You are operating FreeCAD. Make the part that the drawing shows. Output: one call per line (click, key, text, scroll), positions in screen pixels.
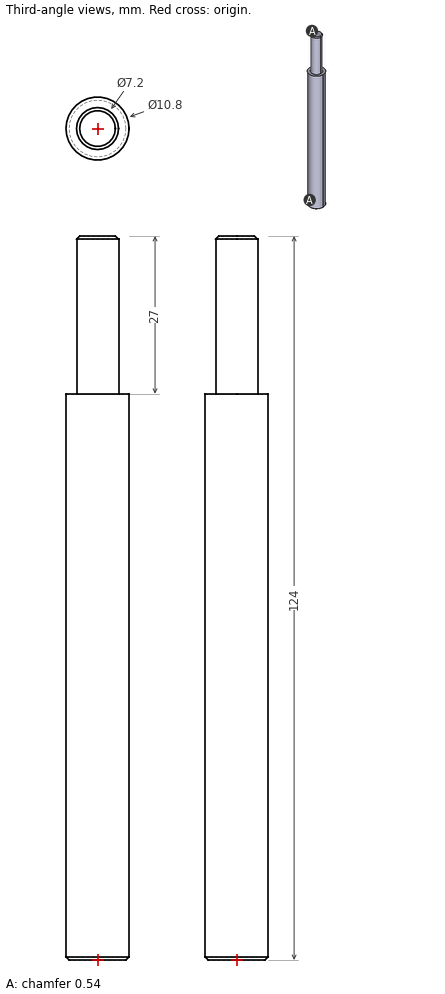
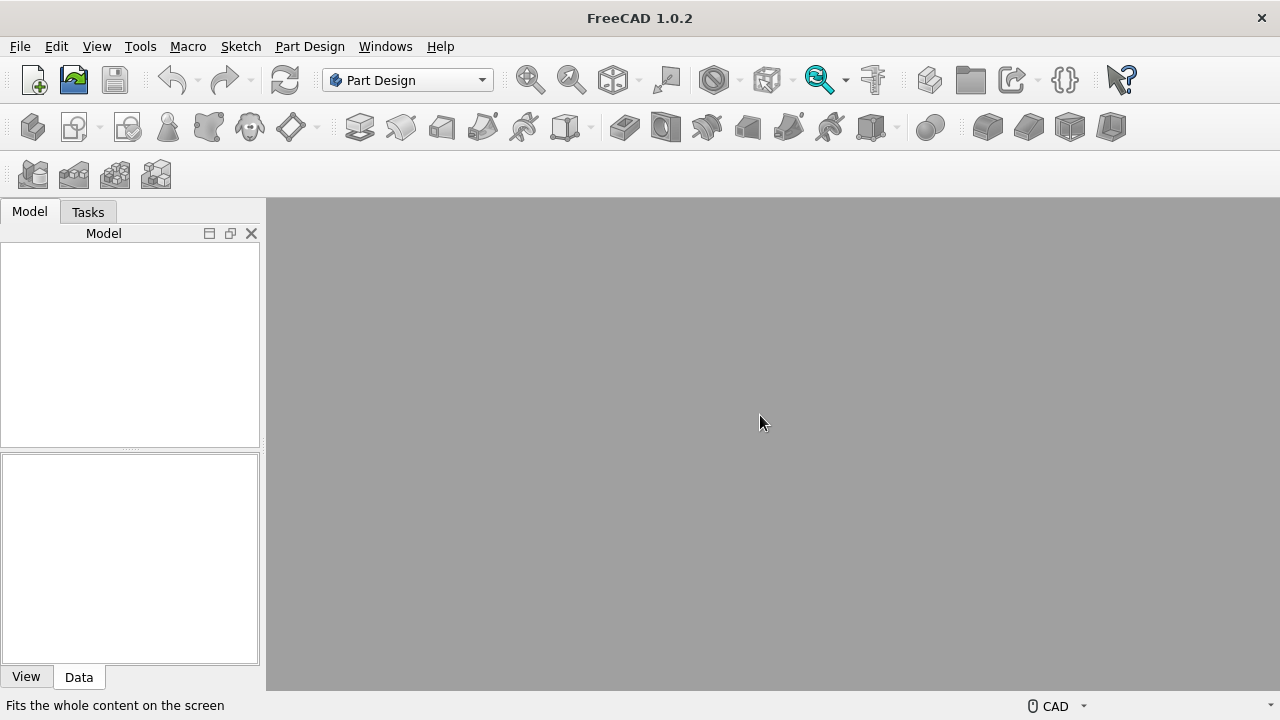
click(33, 80)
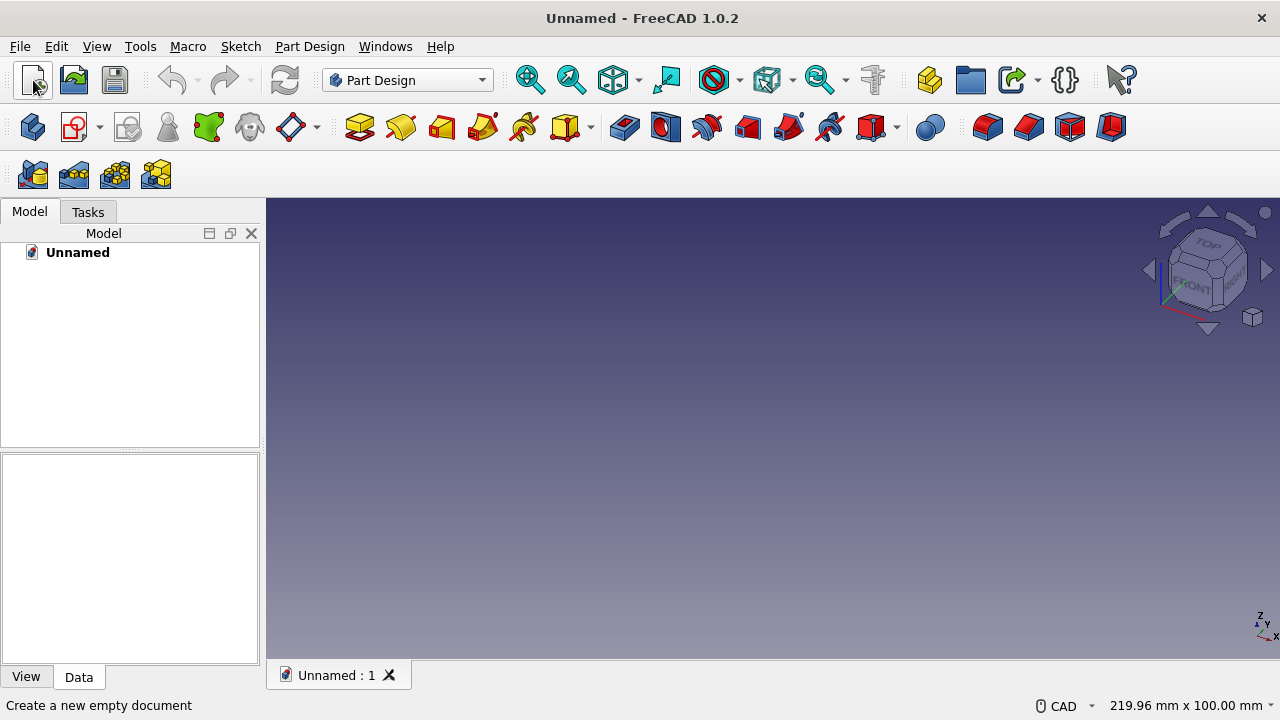
click(74, 128)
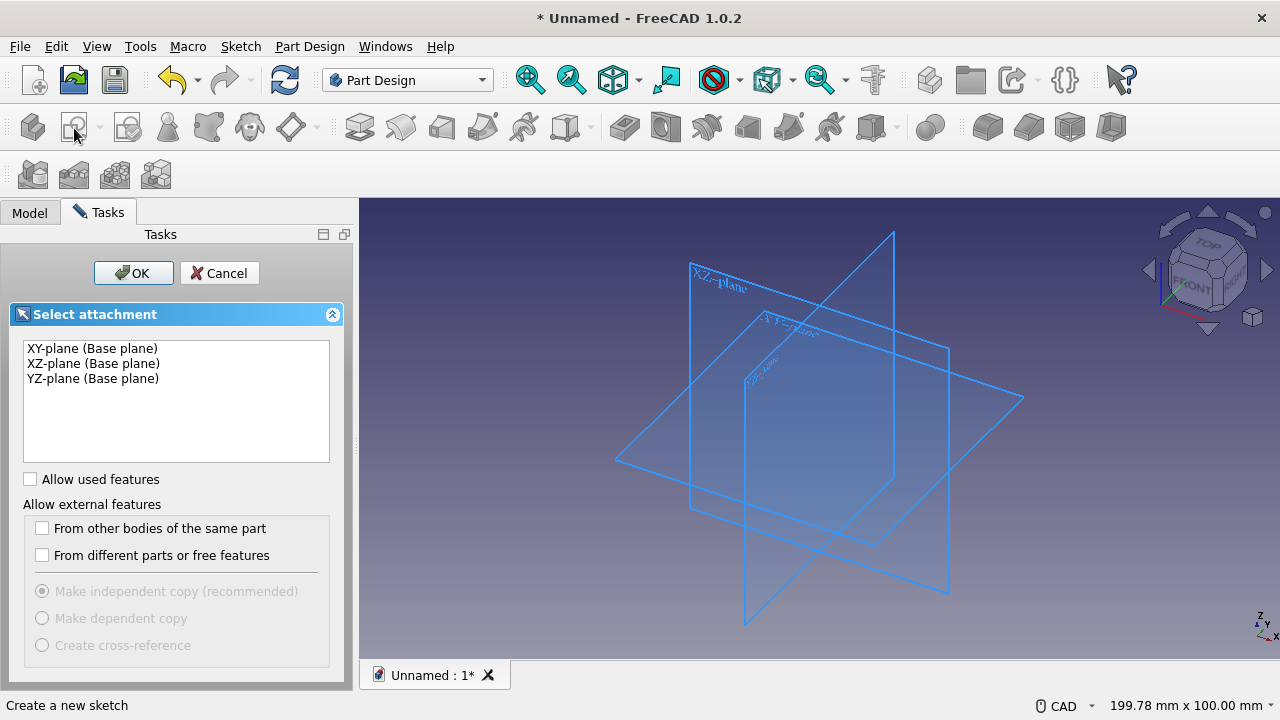
click(84, 348)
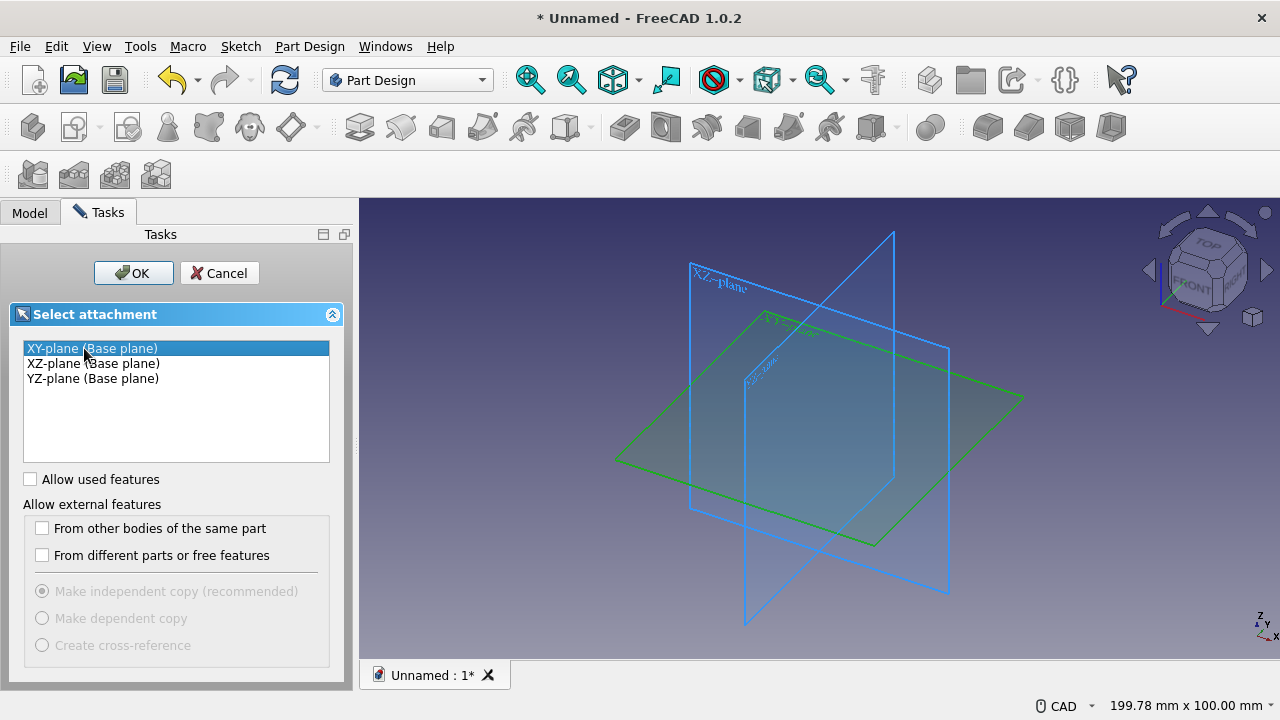
click(134, 273)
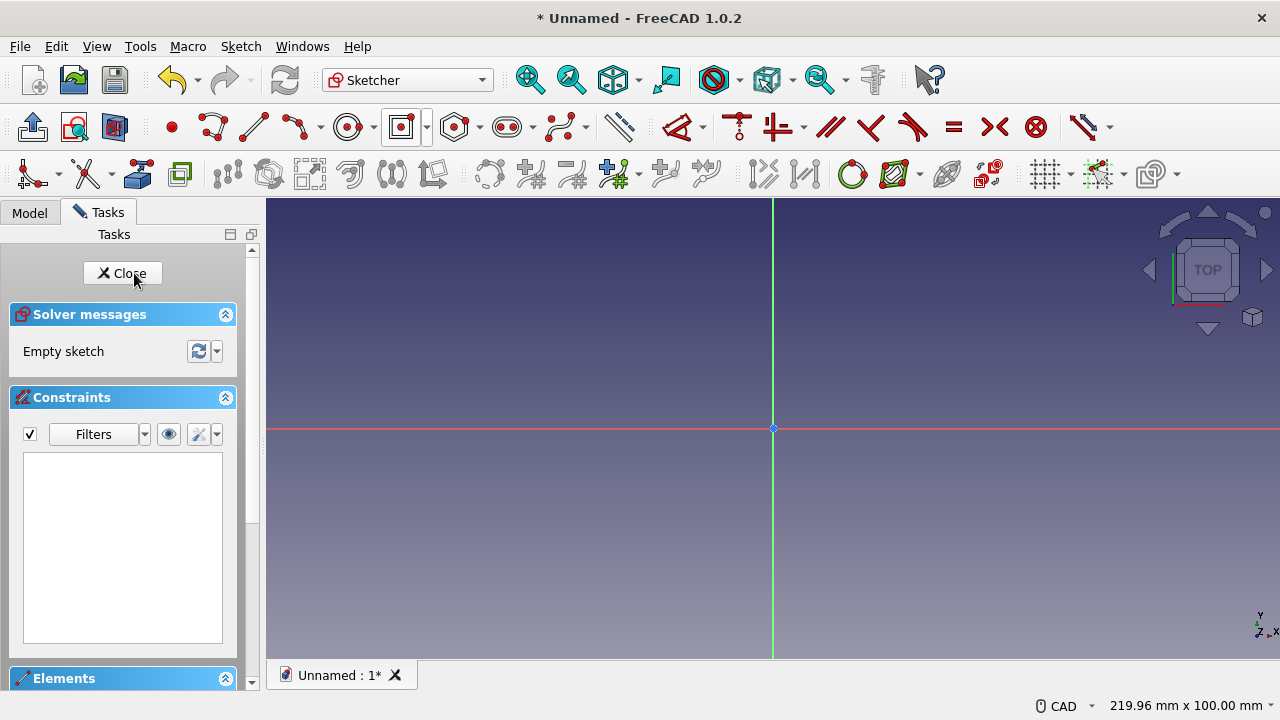
scroll(787, 428, up, 9)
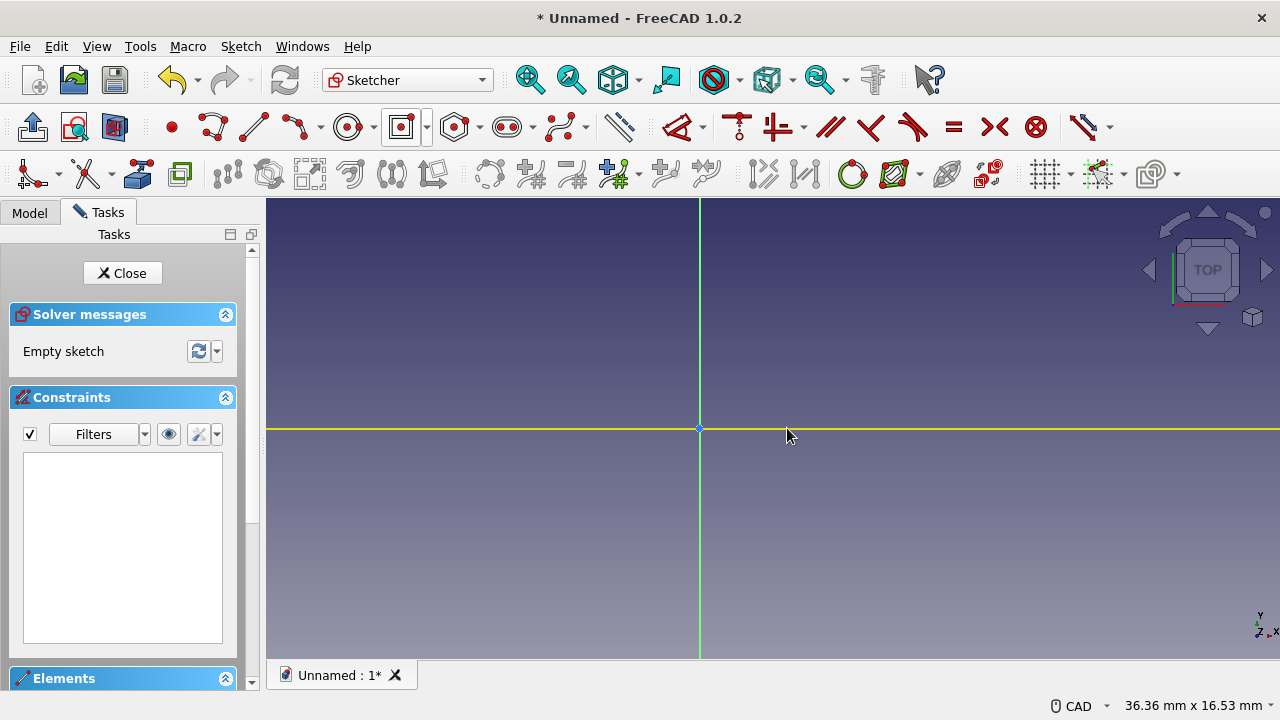
click(348, 128)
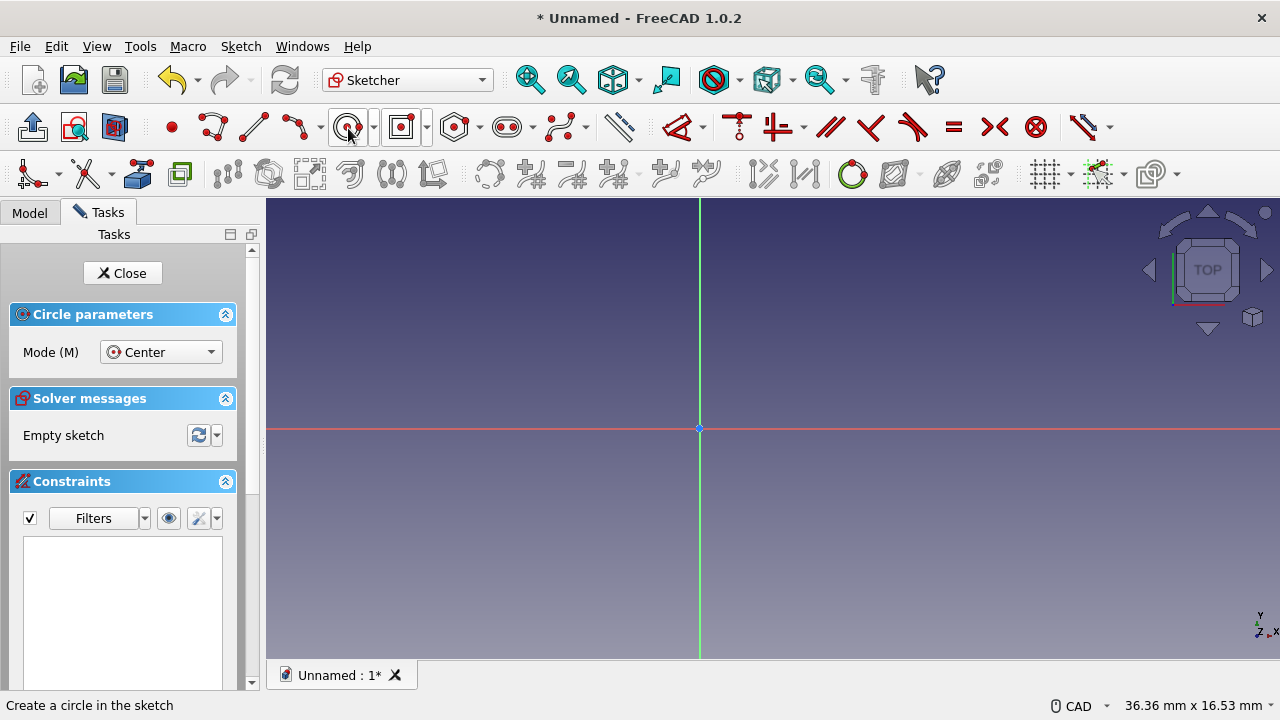
click(700, 428)
click(806, 322)
key(Escape)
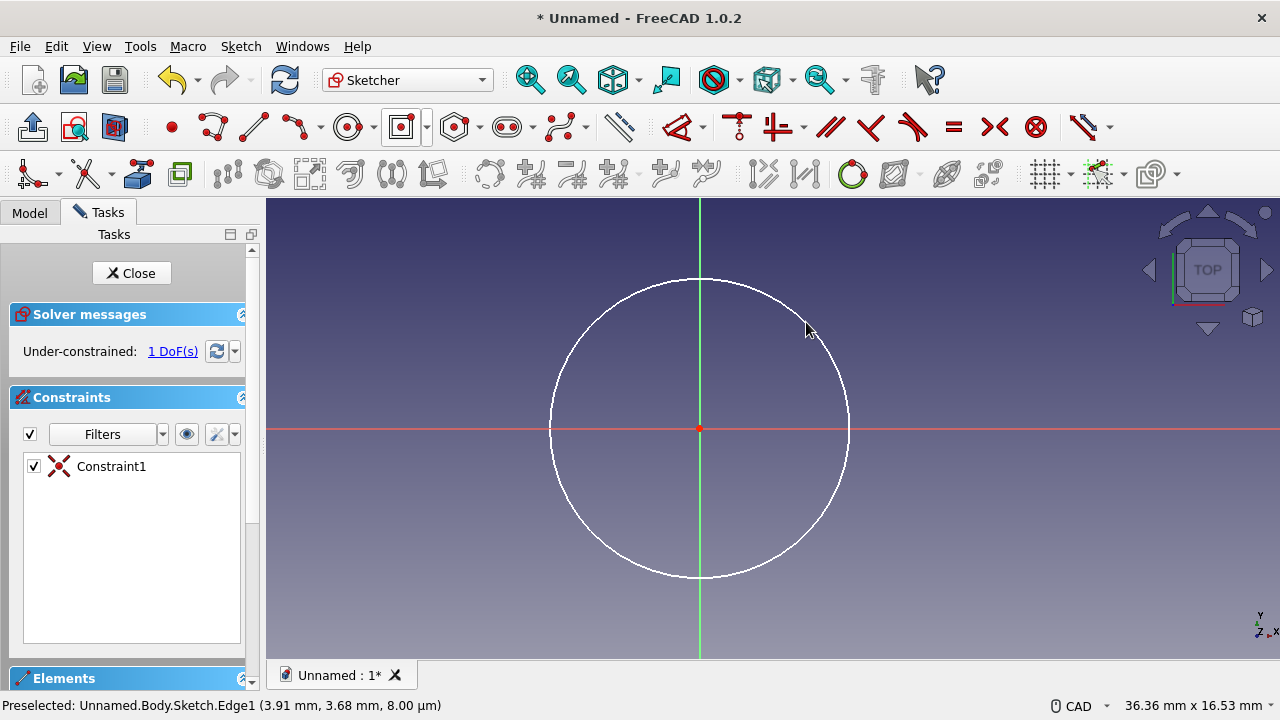
click(676, 128)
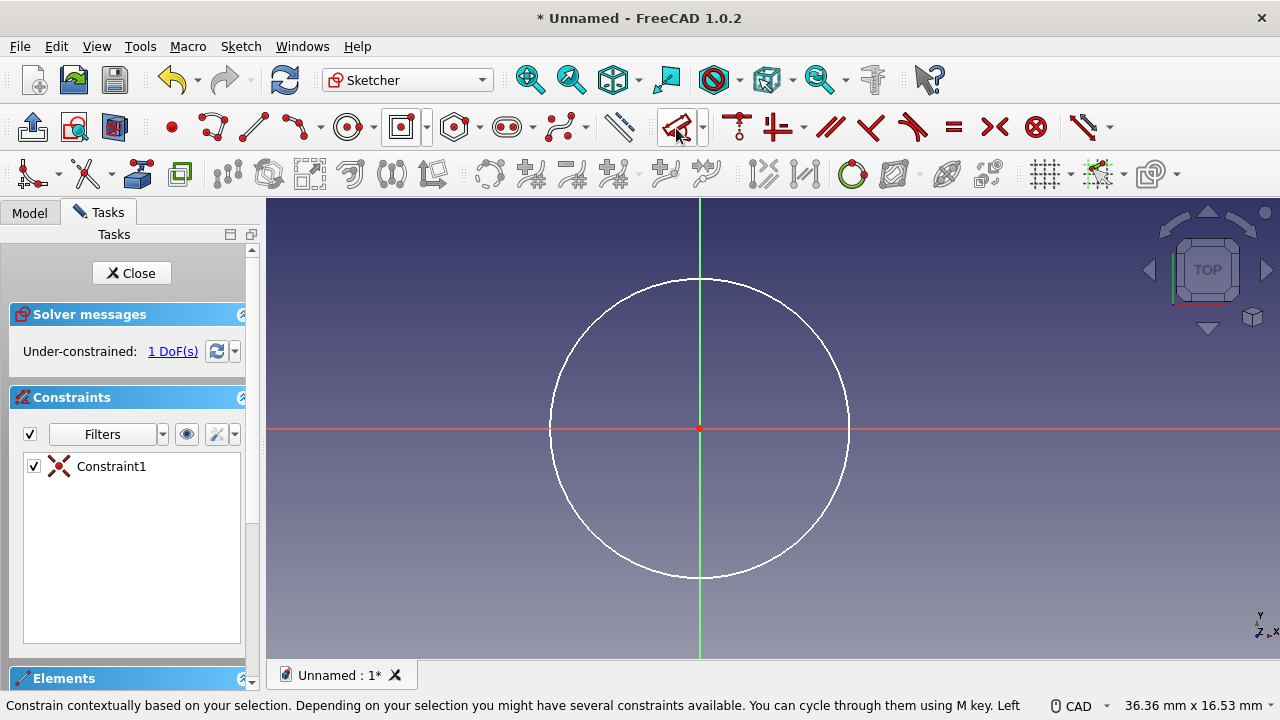
click(805, 322)
click(827, 299)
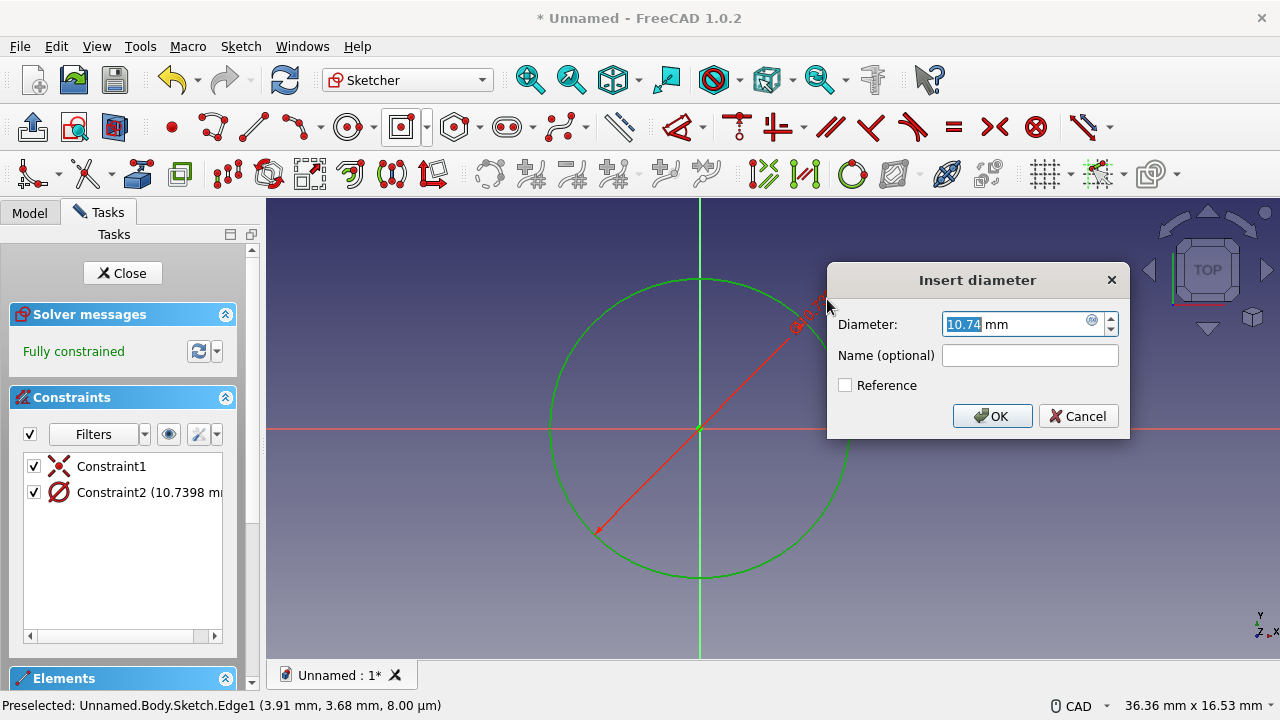
text(10.8)
key(Return)
key(Escape)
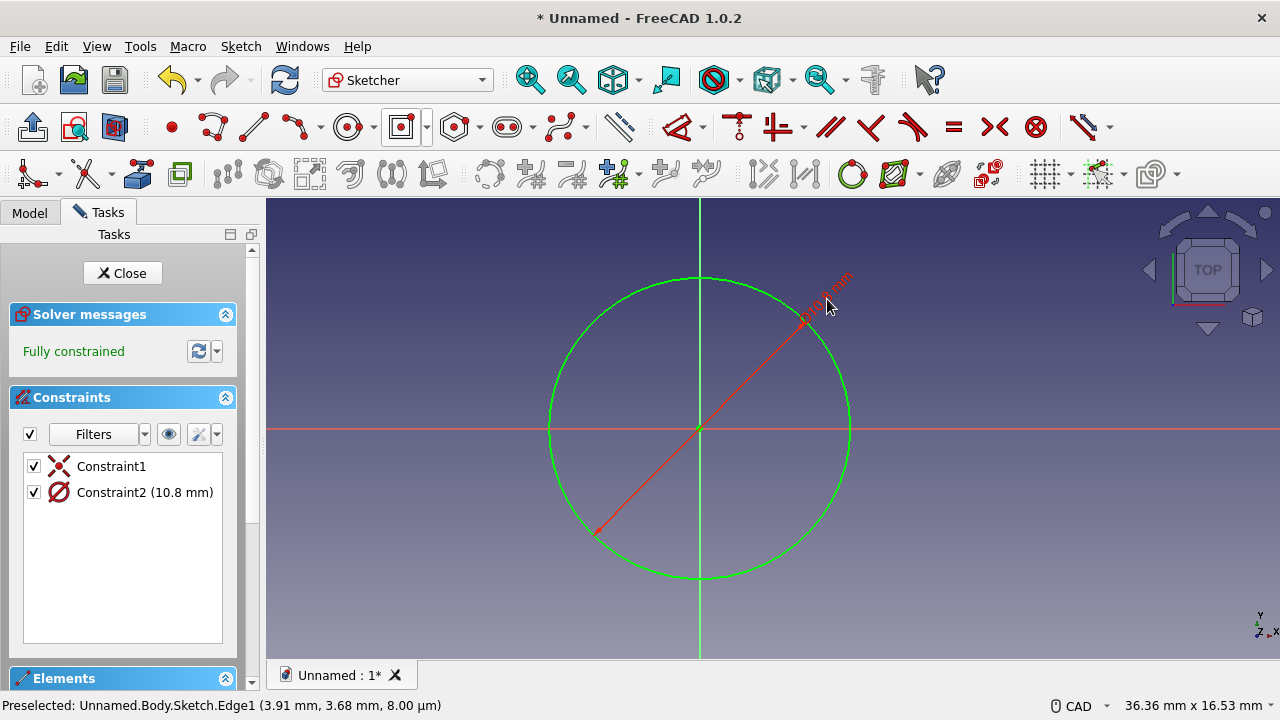
click(123, 273)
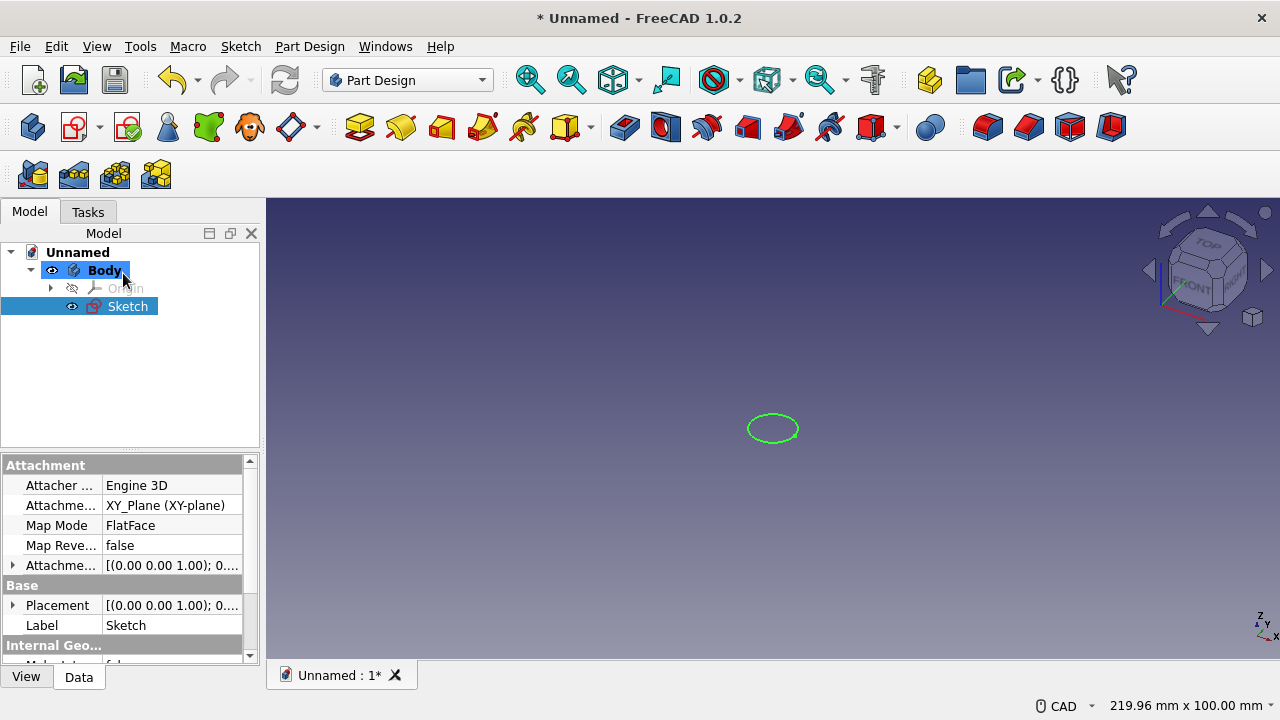
click(360, 128)